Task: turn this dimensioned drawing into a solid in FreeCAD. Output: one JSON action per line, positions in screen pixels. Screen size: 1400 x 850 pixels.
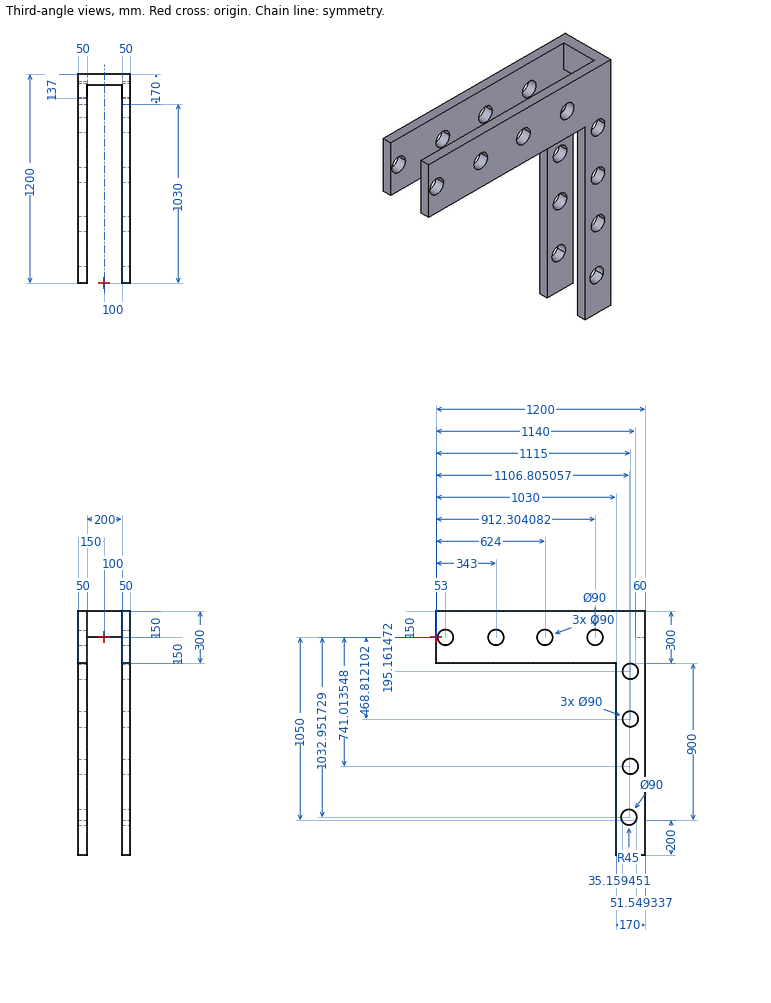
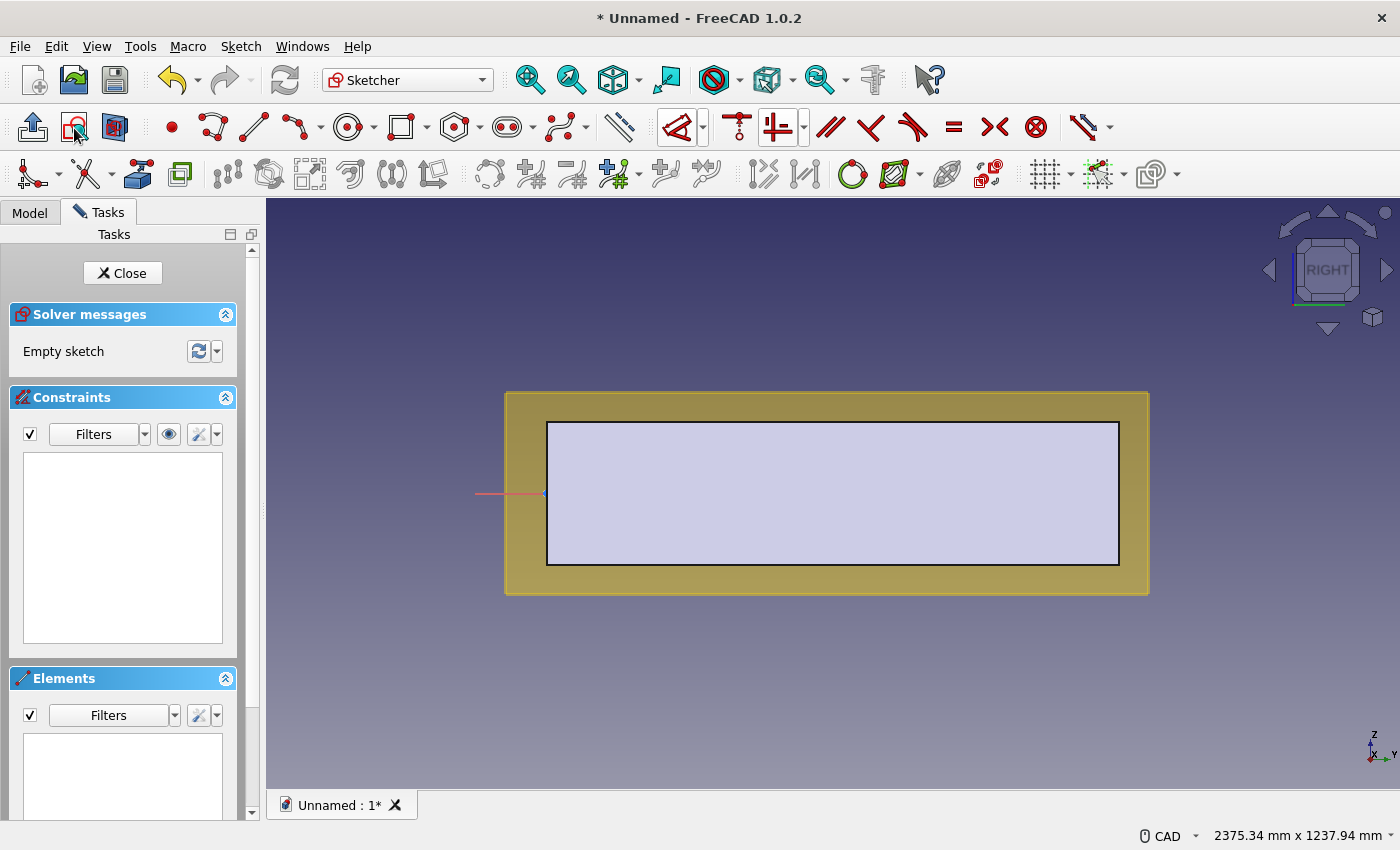
{"action": "left_click", "coordinate": [115, 128]}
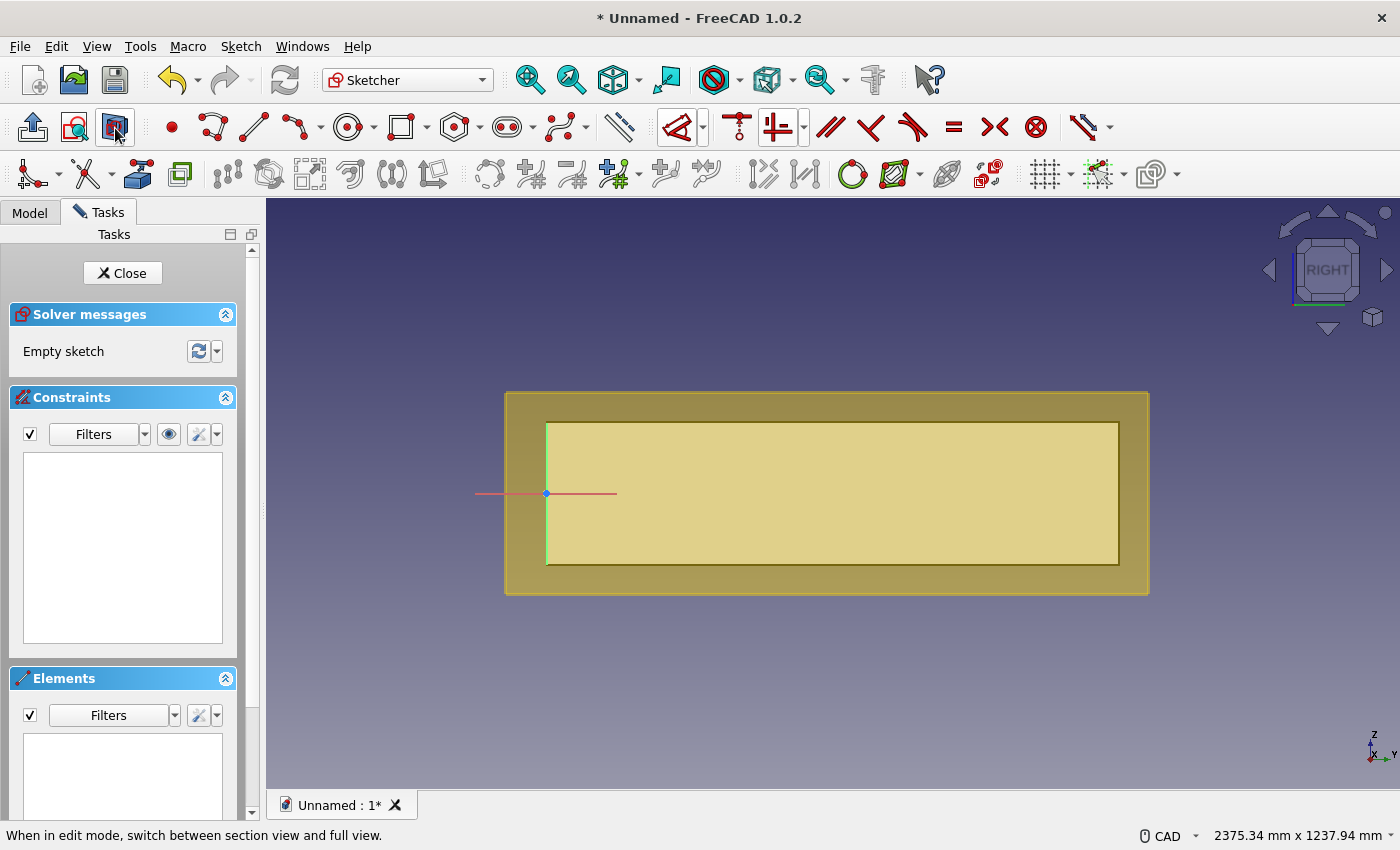
{"action": "scroll", "coordinate": [1235, 494], "scroll_direction": "up", "scroll_amount": 5}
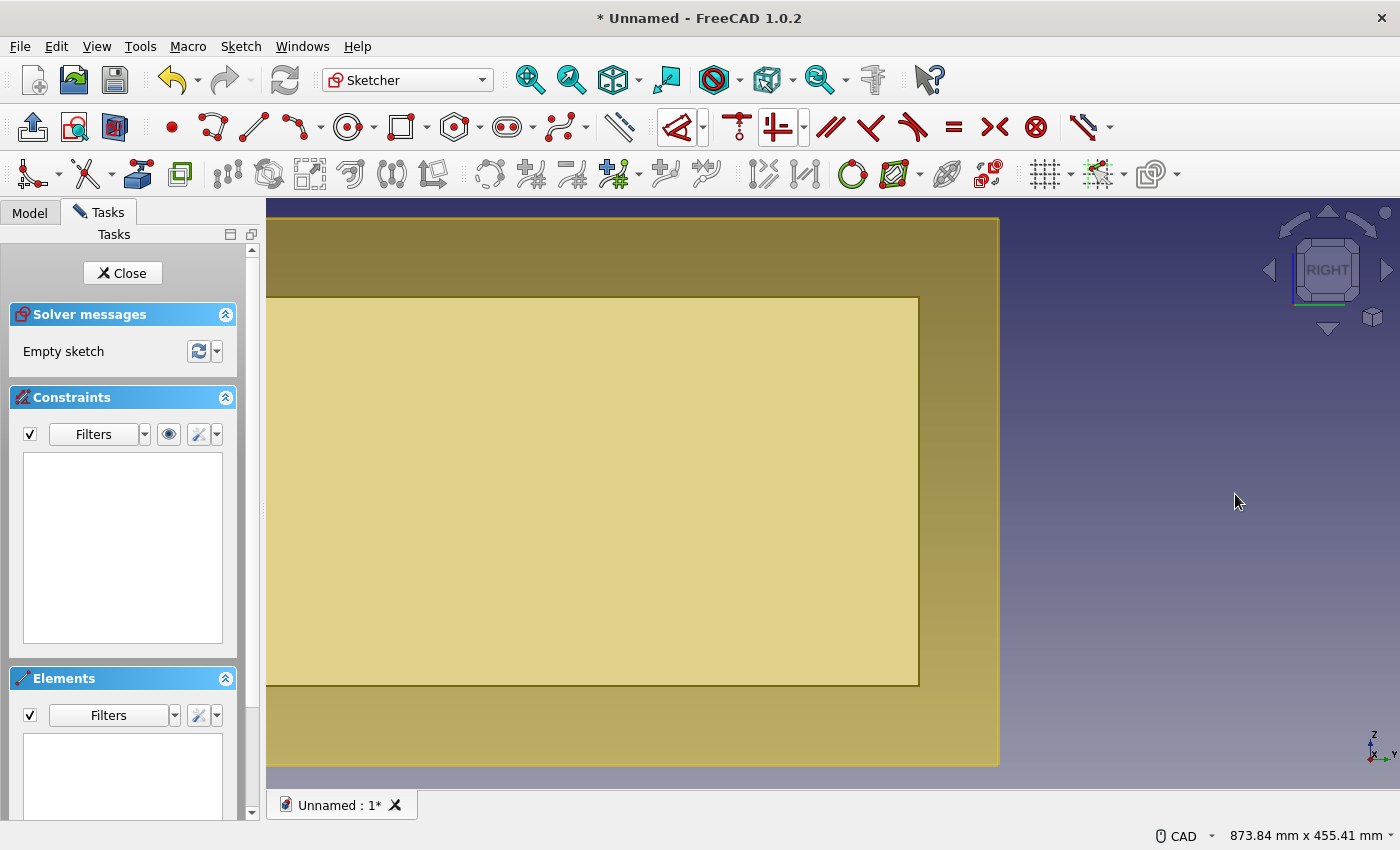
{"action": "left_click", "coordinate": [400, 128]}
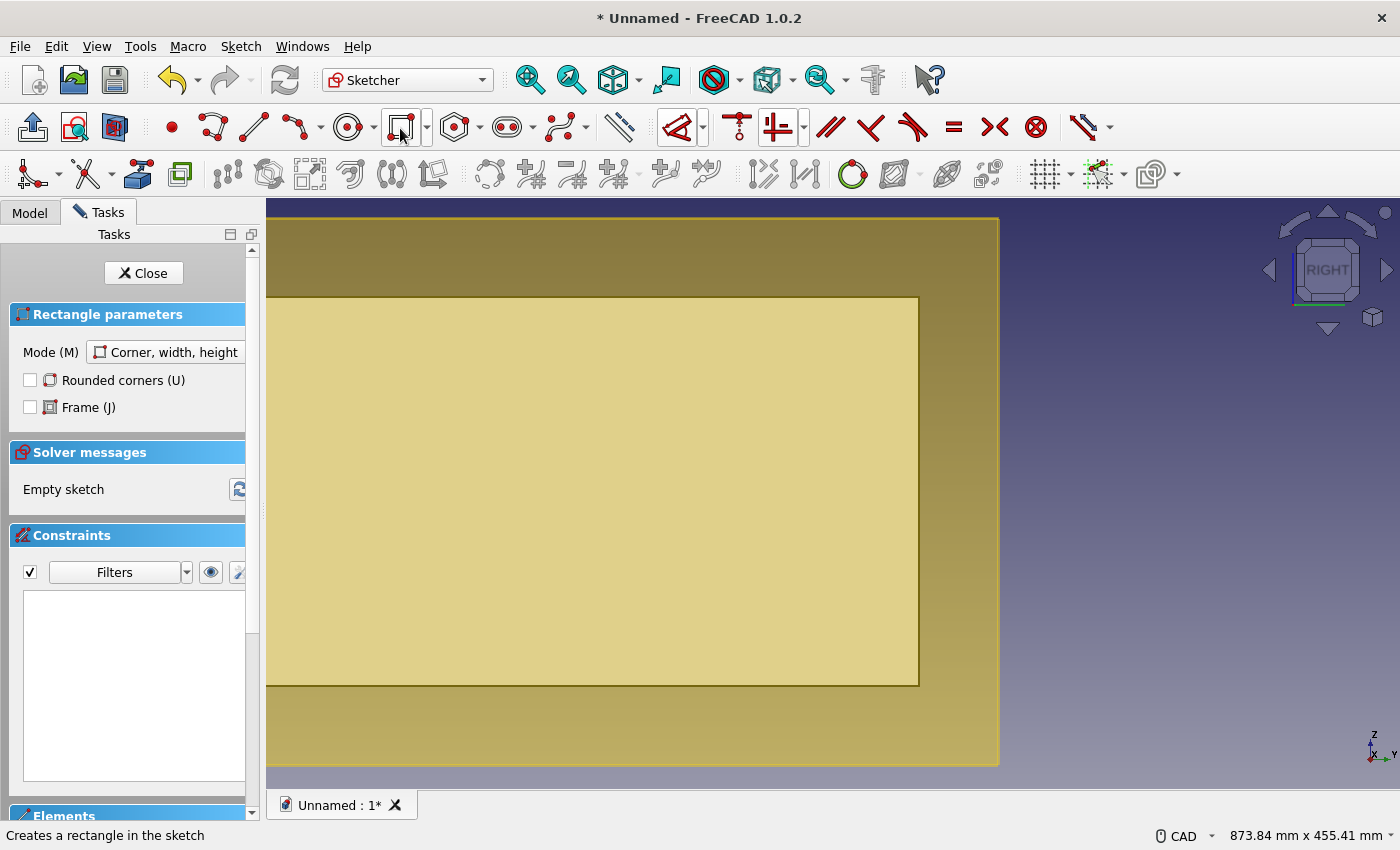
{"action": "left_click", "coordinate": [842, 297]}
{"action": "left_click", "coordinate": [919, 686]}
{"action": "key", "text": "Escape"}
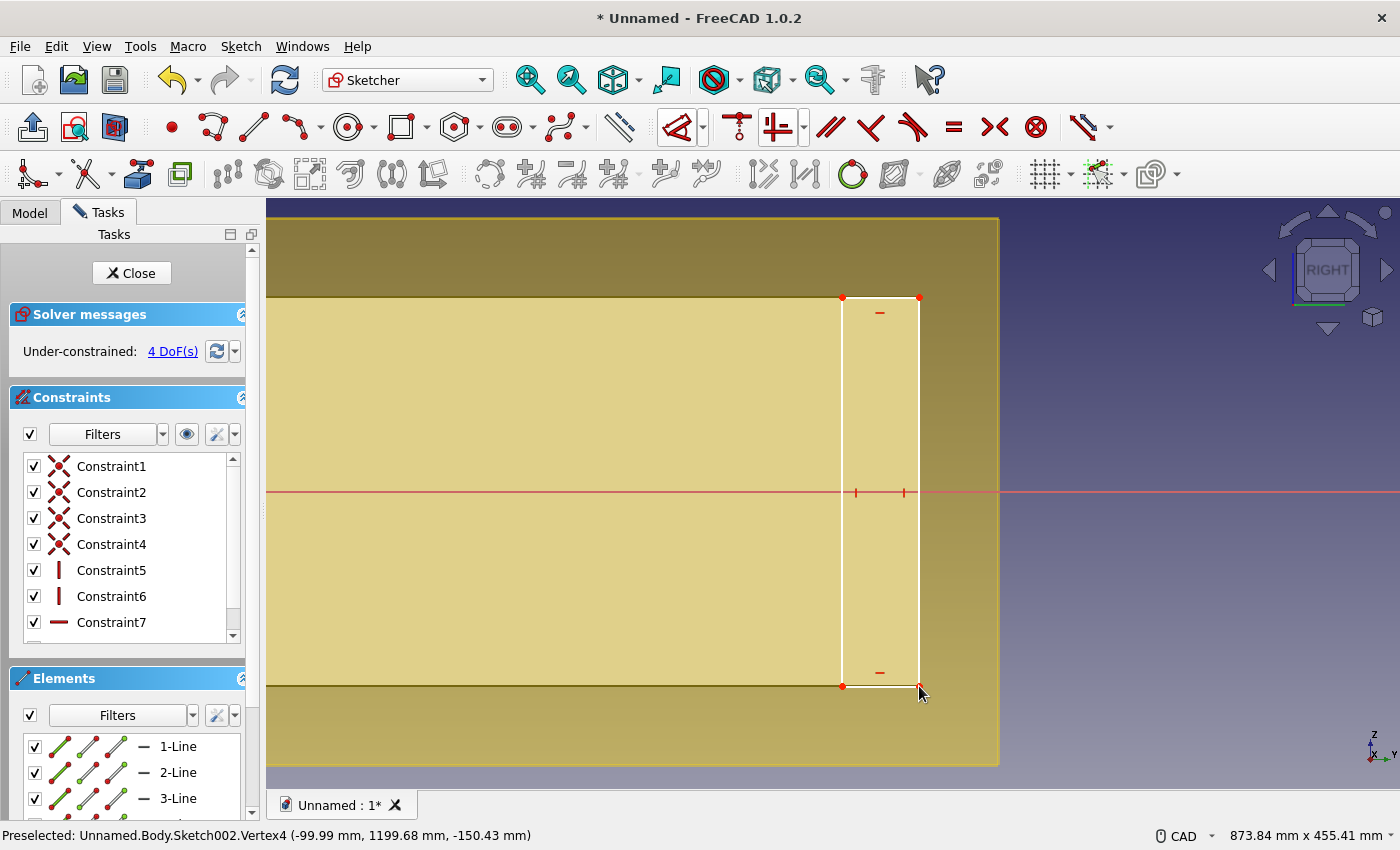
{"action": "left_click", "coordinate": [865, 687]}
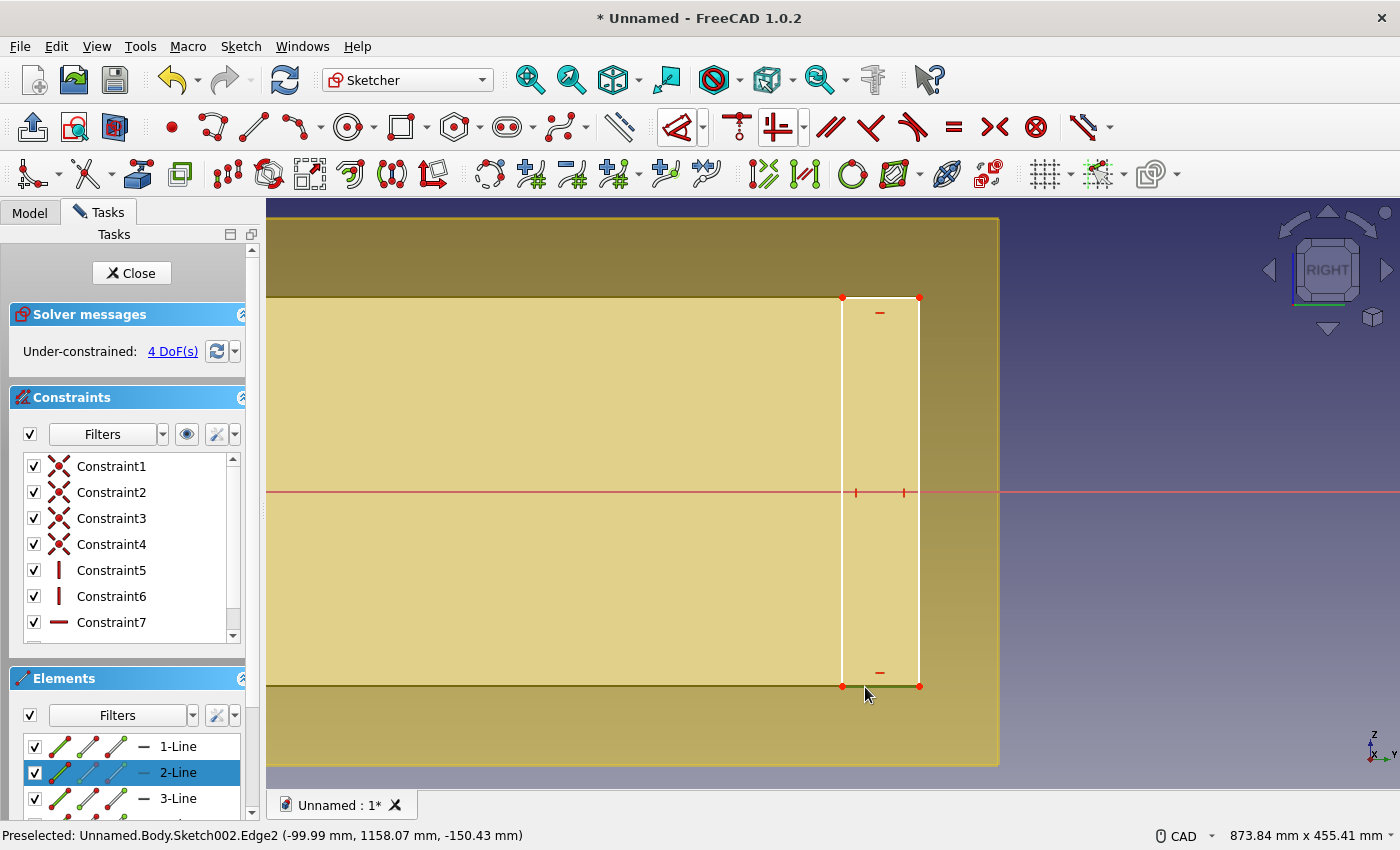
{"action": "key", "text": "l"}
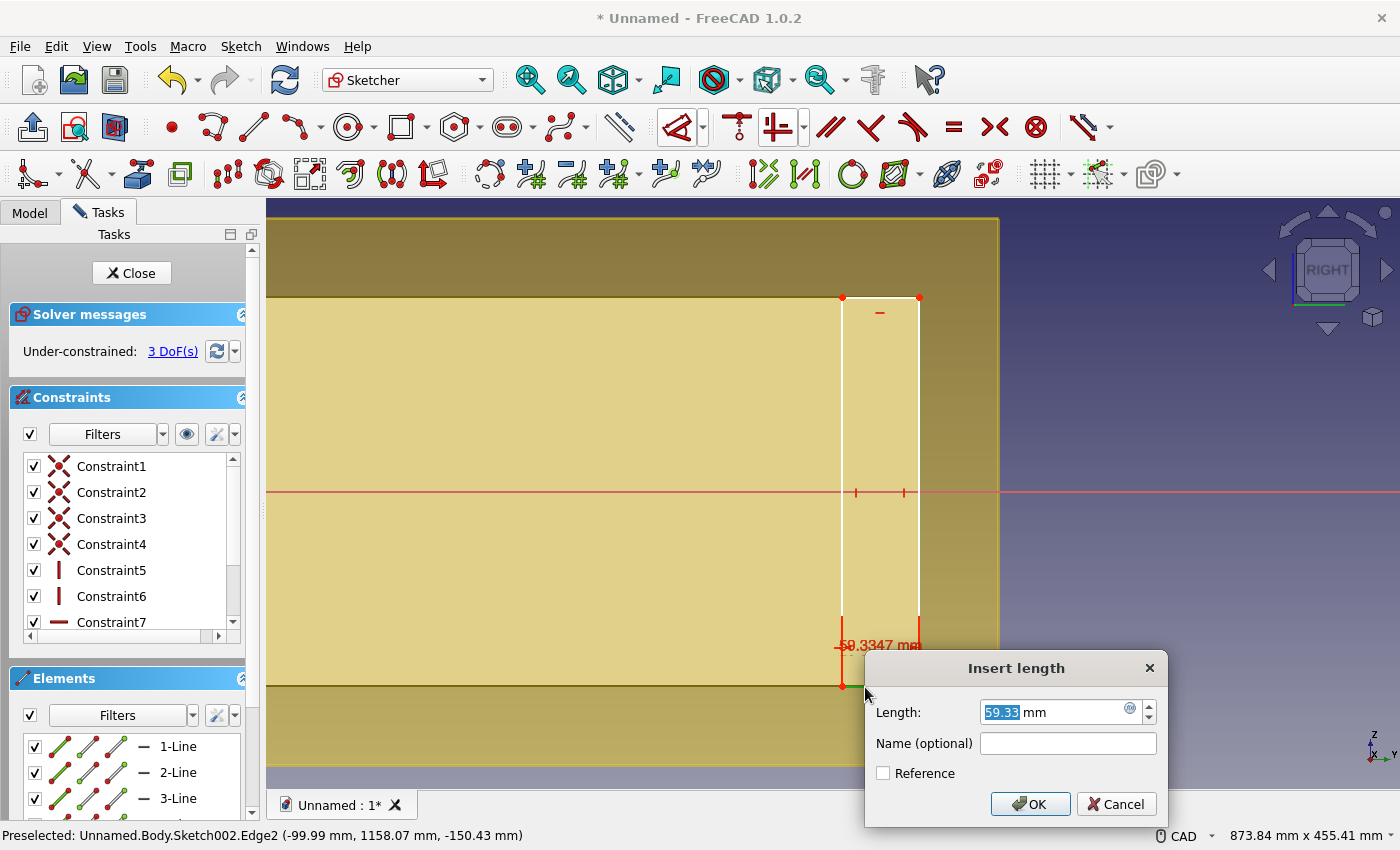
{"action": "type", "text": "60"}
{"action": "key", "text": "Return"}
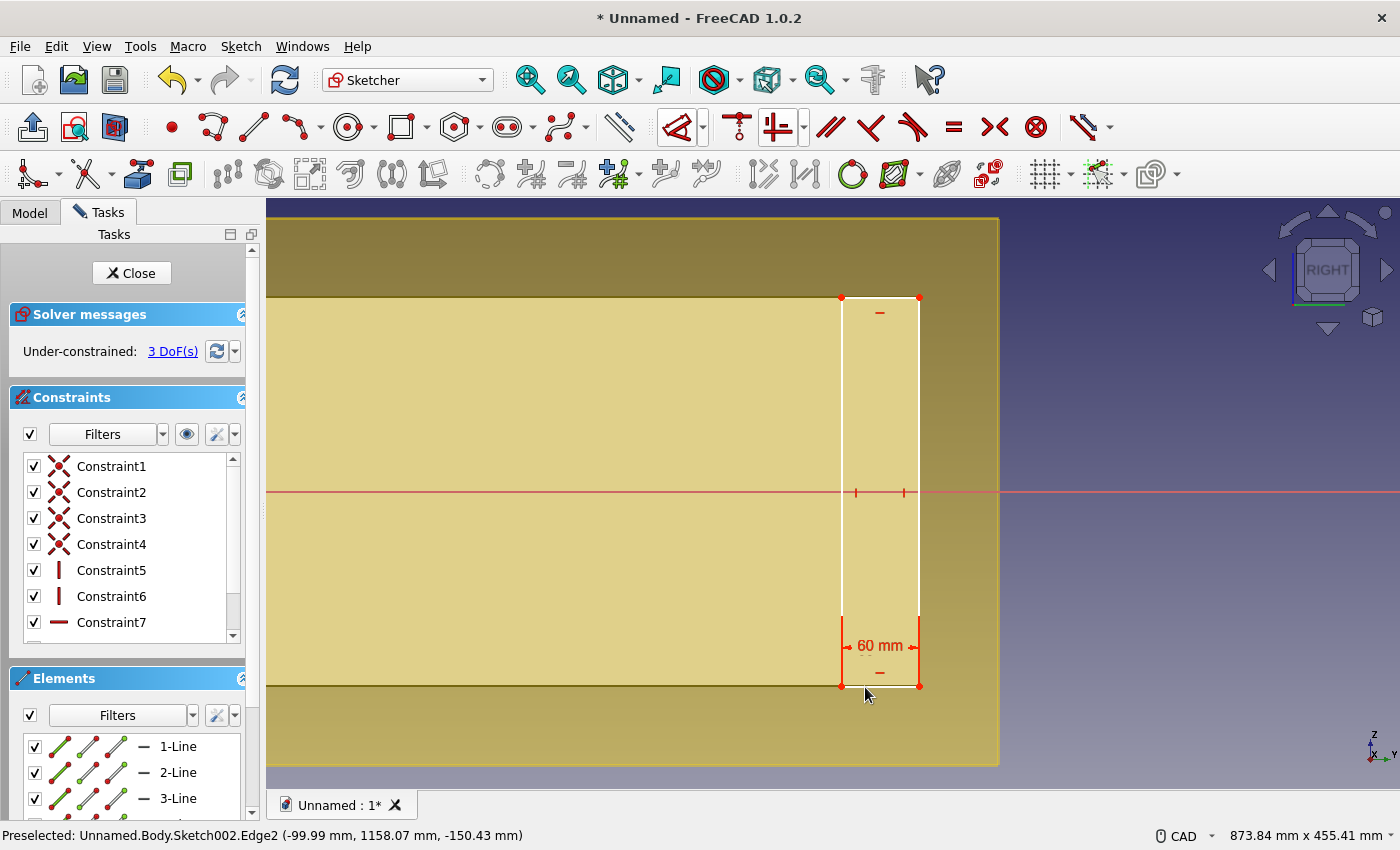
{"action": "left_click", "coordinate": [842, 415]}